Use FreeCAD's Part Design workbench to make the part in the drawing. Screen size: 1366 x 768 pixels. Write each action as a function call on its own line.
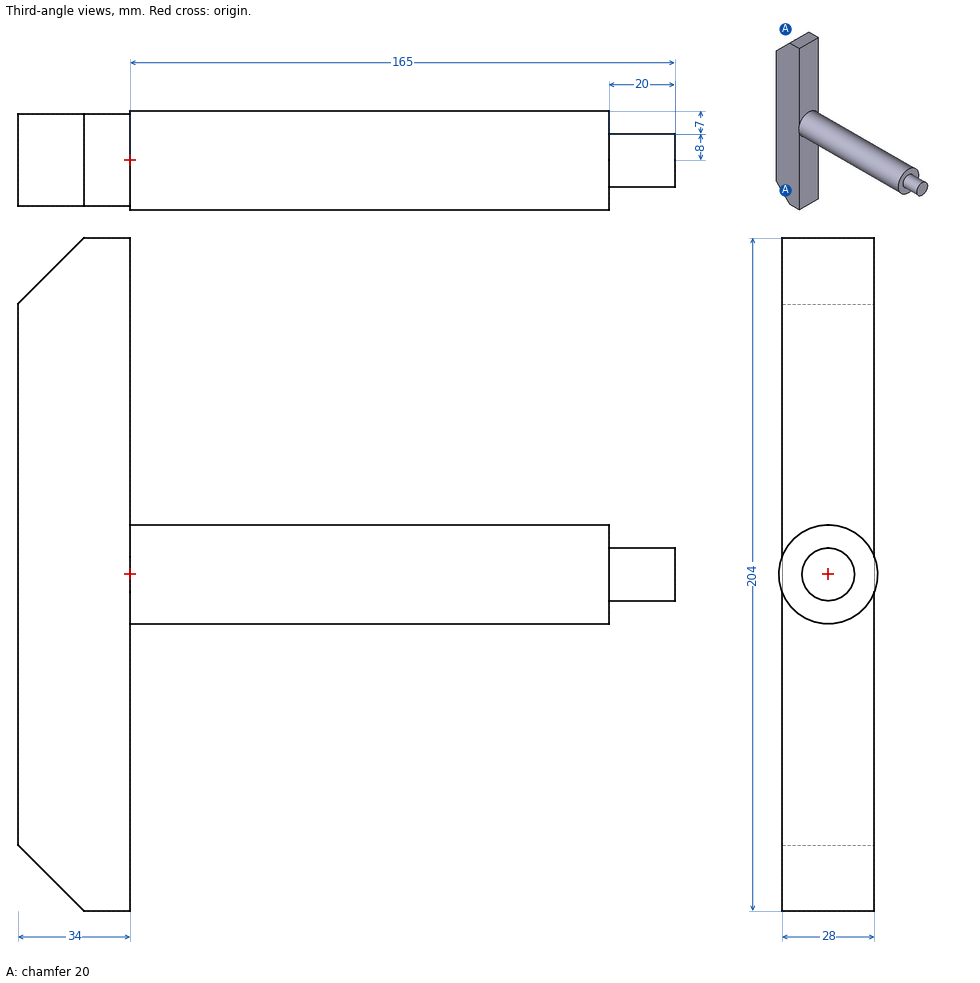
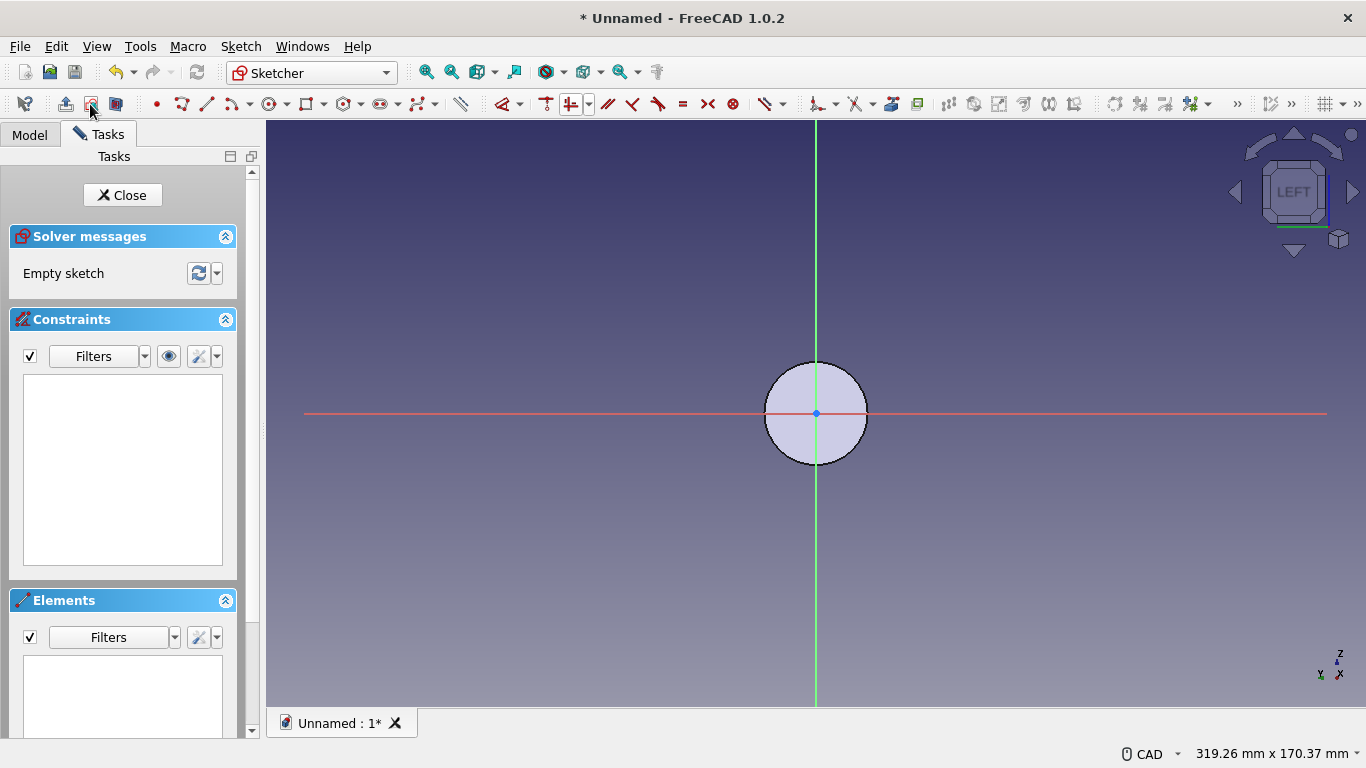
scroll(664, 414, down, 3)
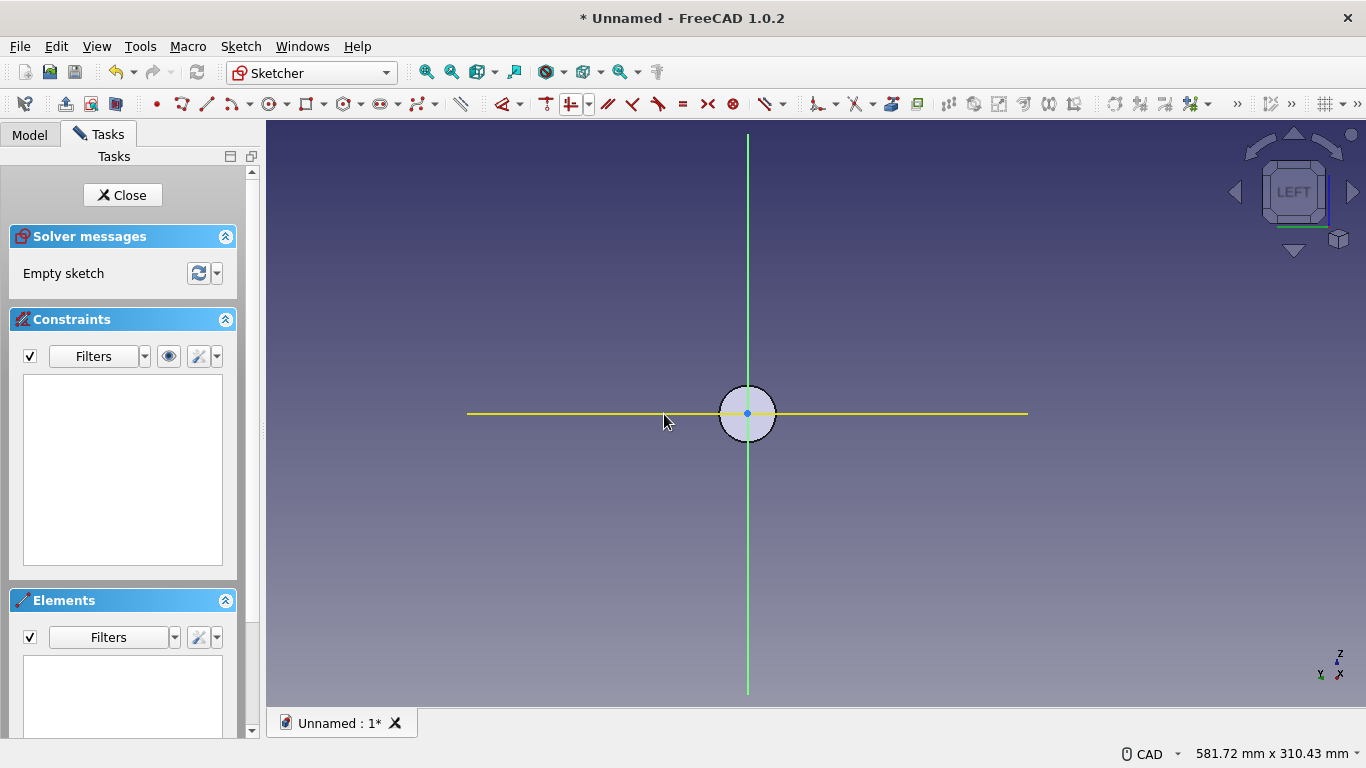
key(g)
key(v)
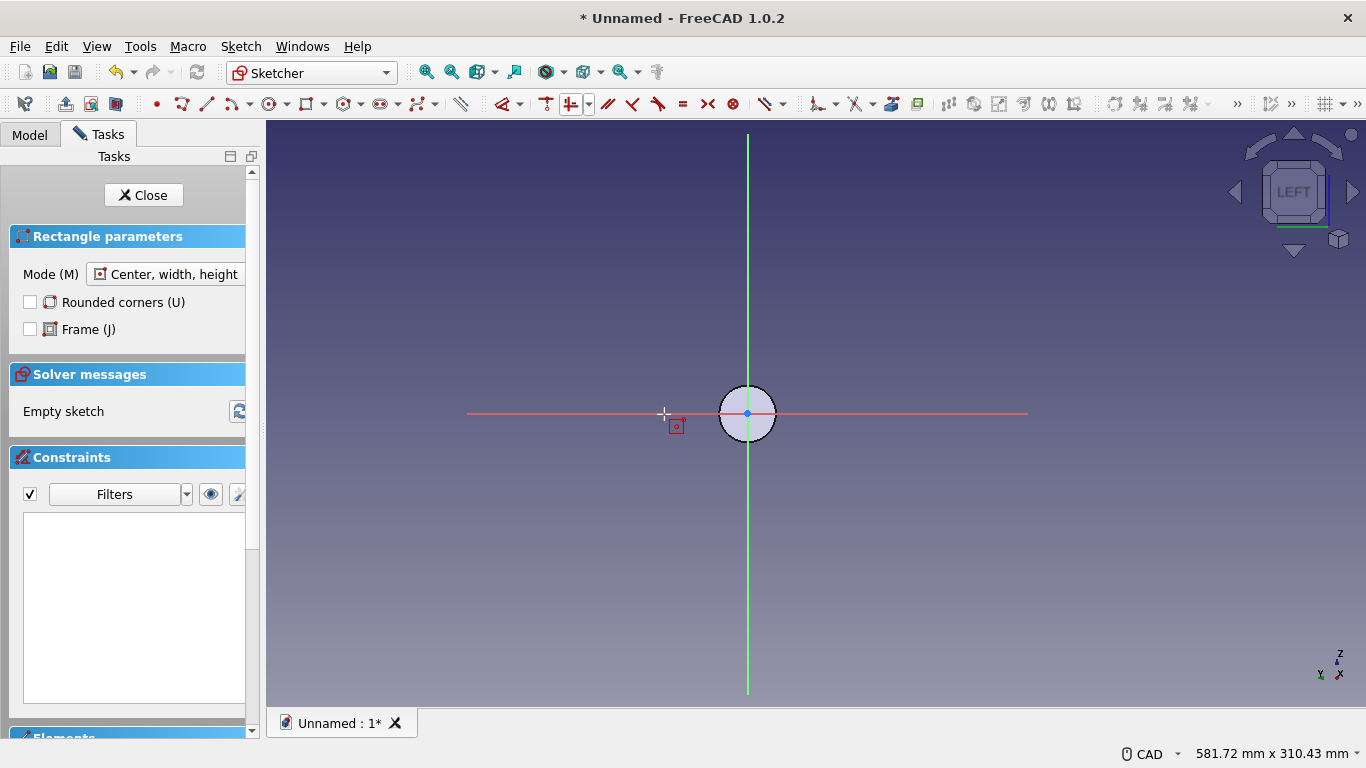
click(748, 414)
click(774, 221)
key(Escape)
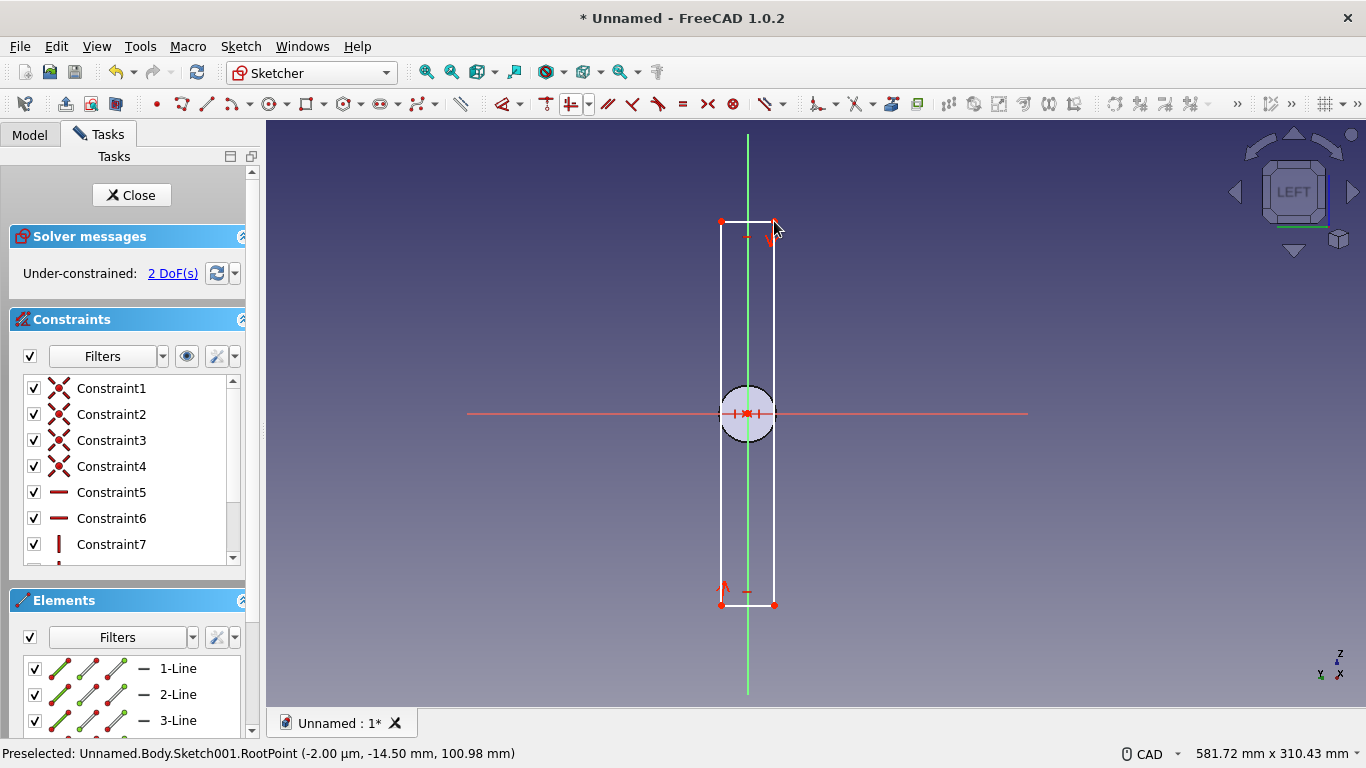
click(502, 104)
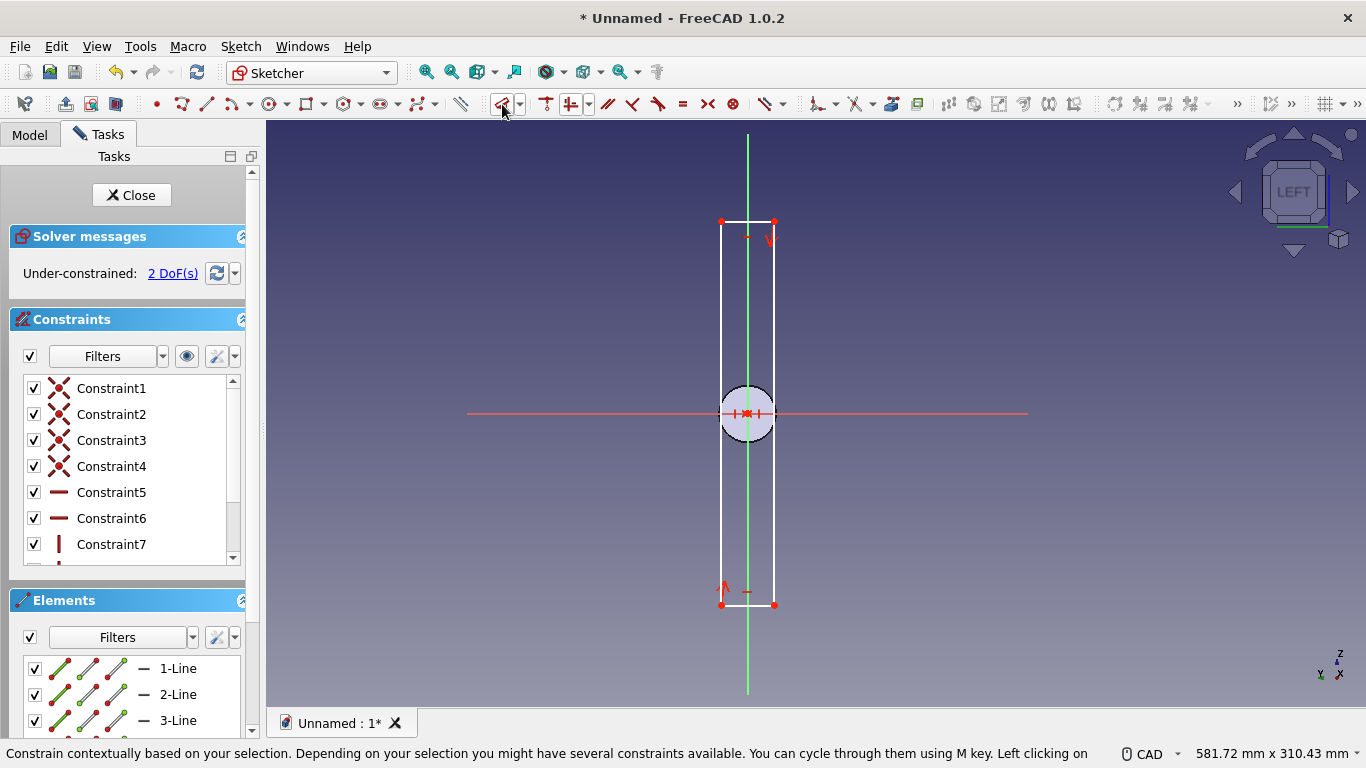
scroll(737, 606, up, 2)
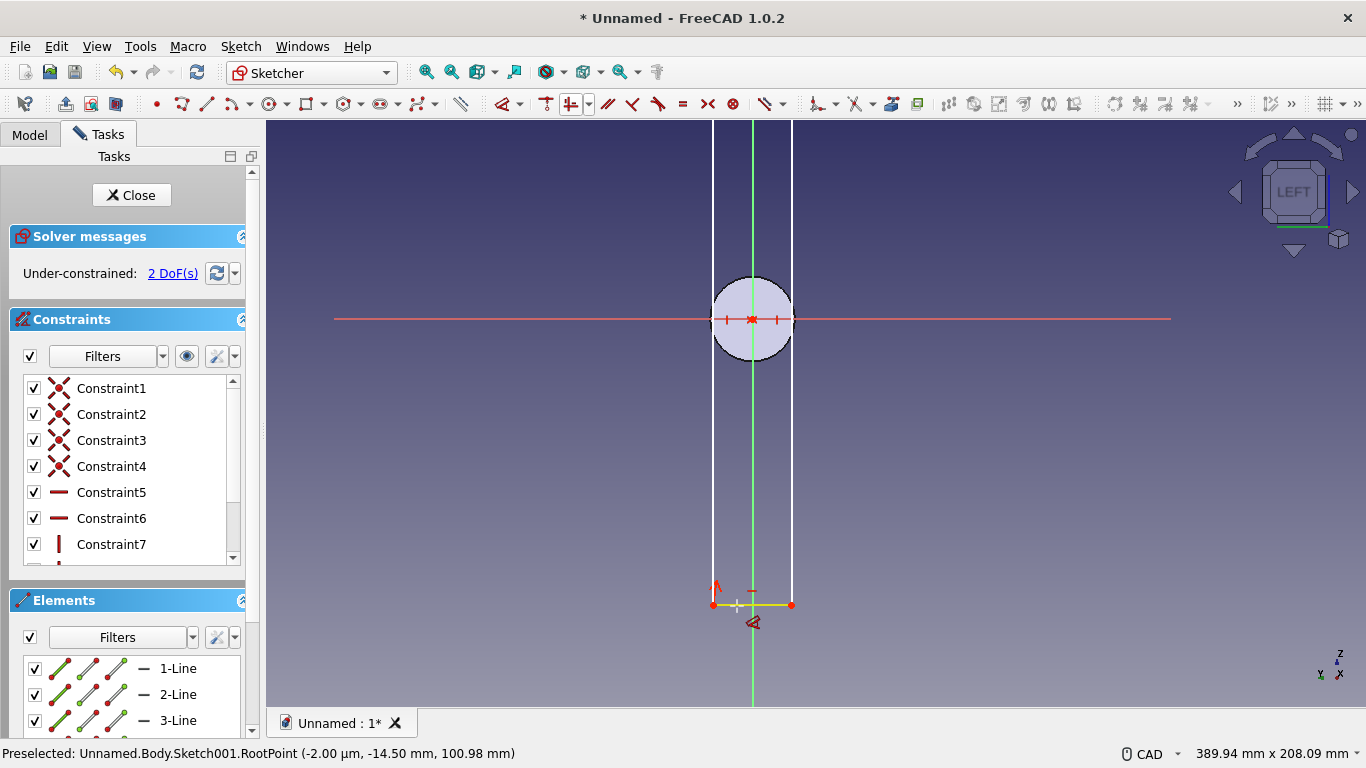
click(737, 605)
click(734, 639)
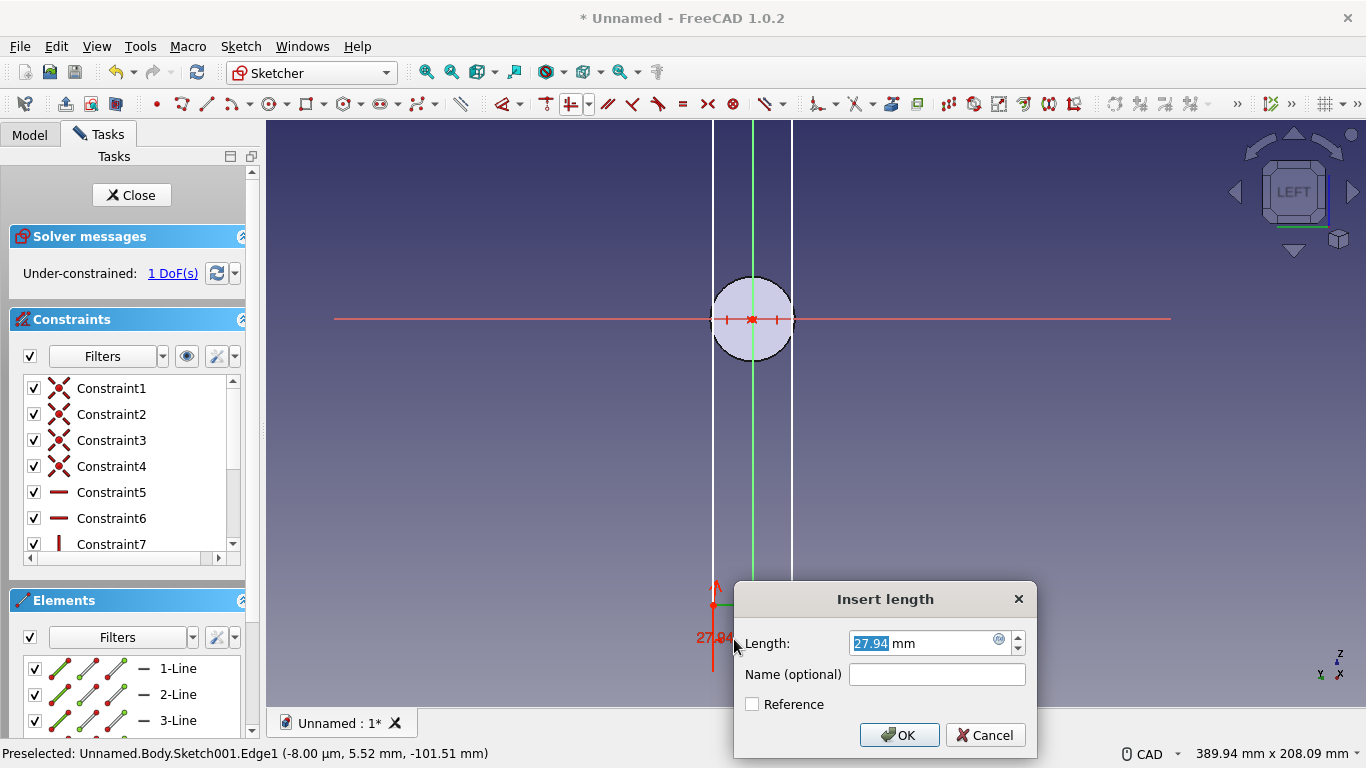
text(28)
key(Return)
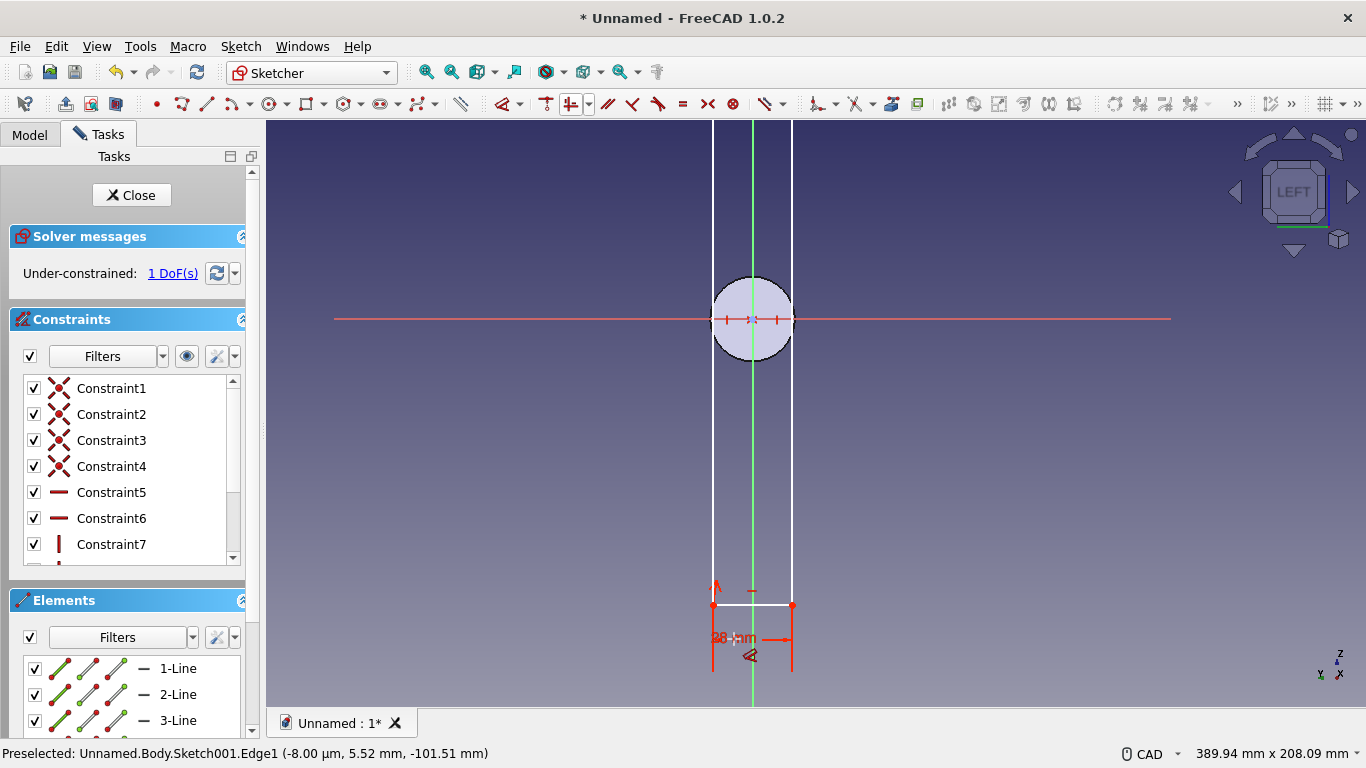
click(792, 434)
click(826, 377)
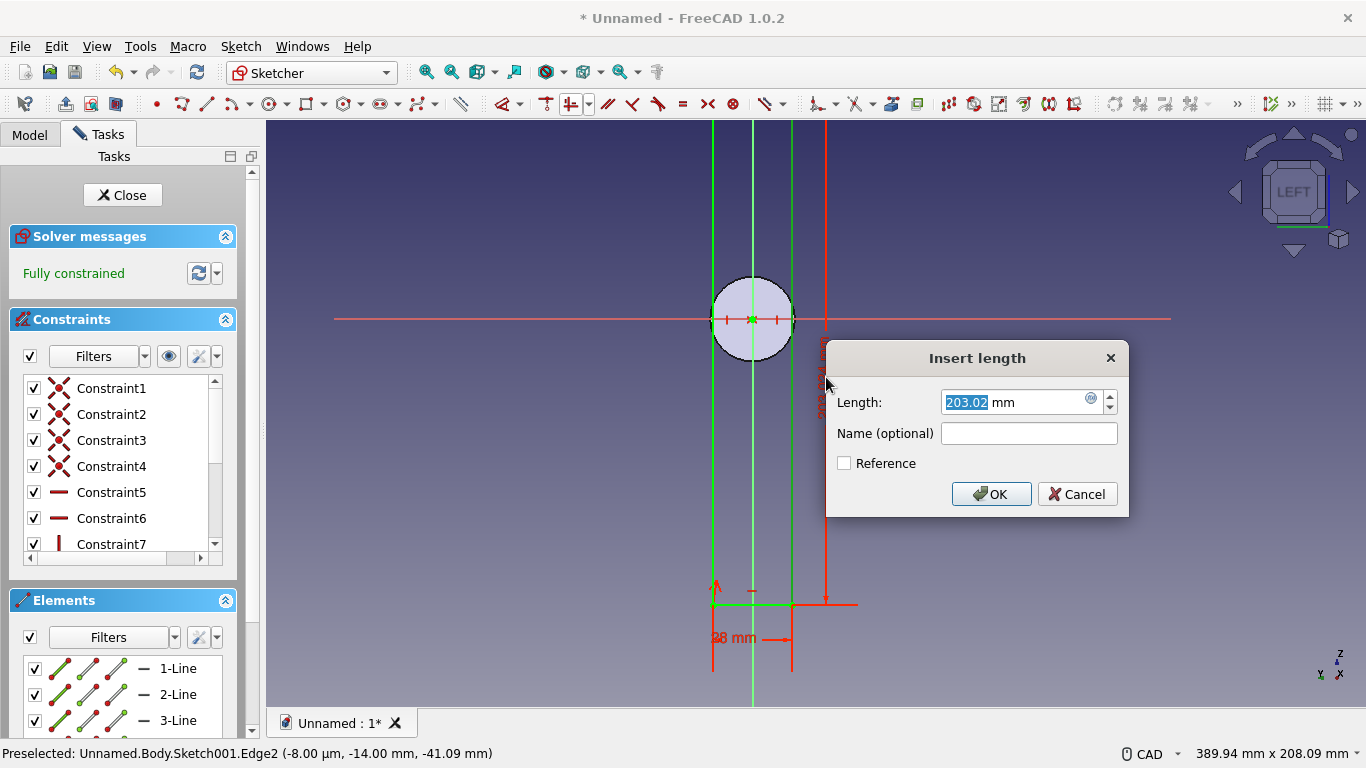
text(204)
key(Return)
key(Escape)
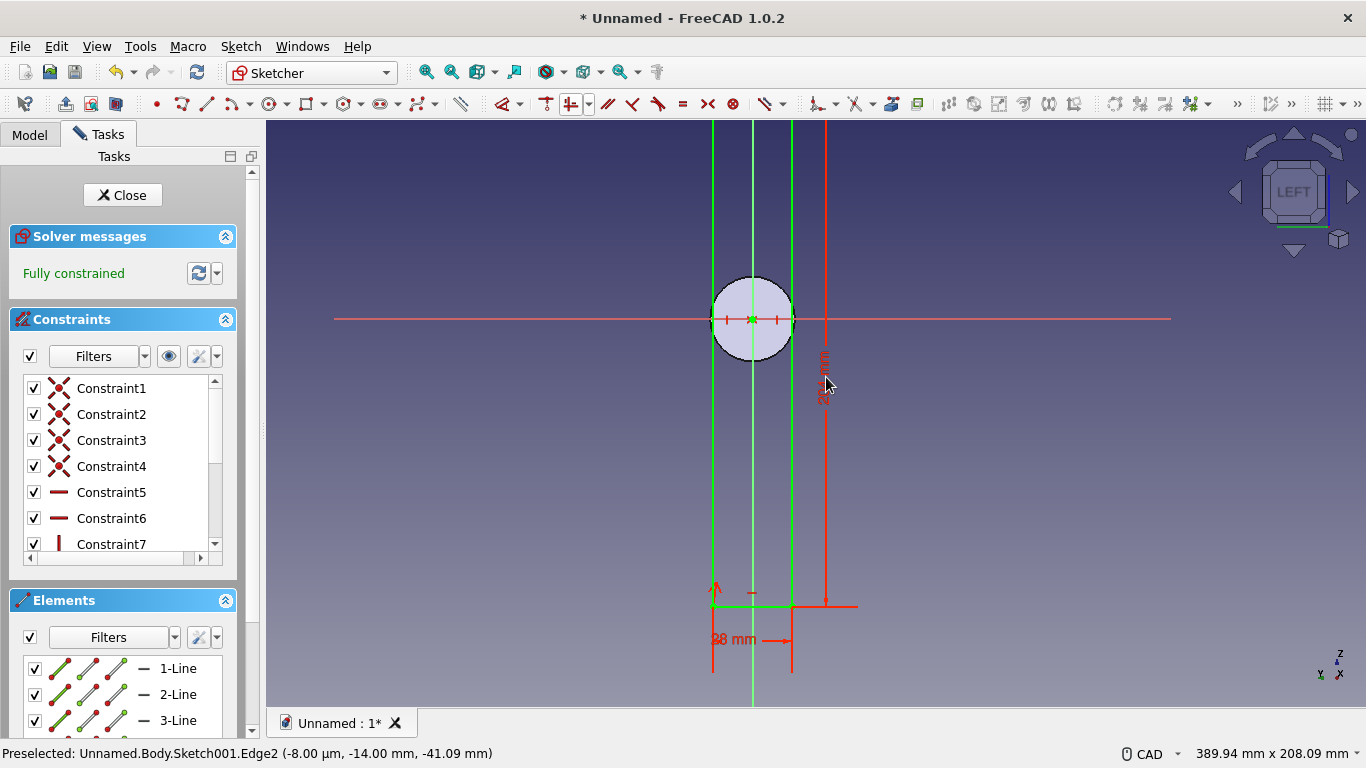
click(123, 195)